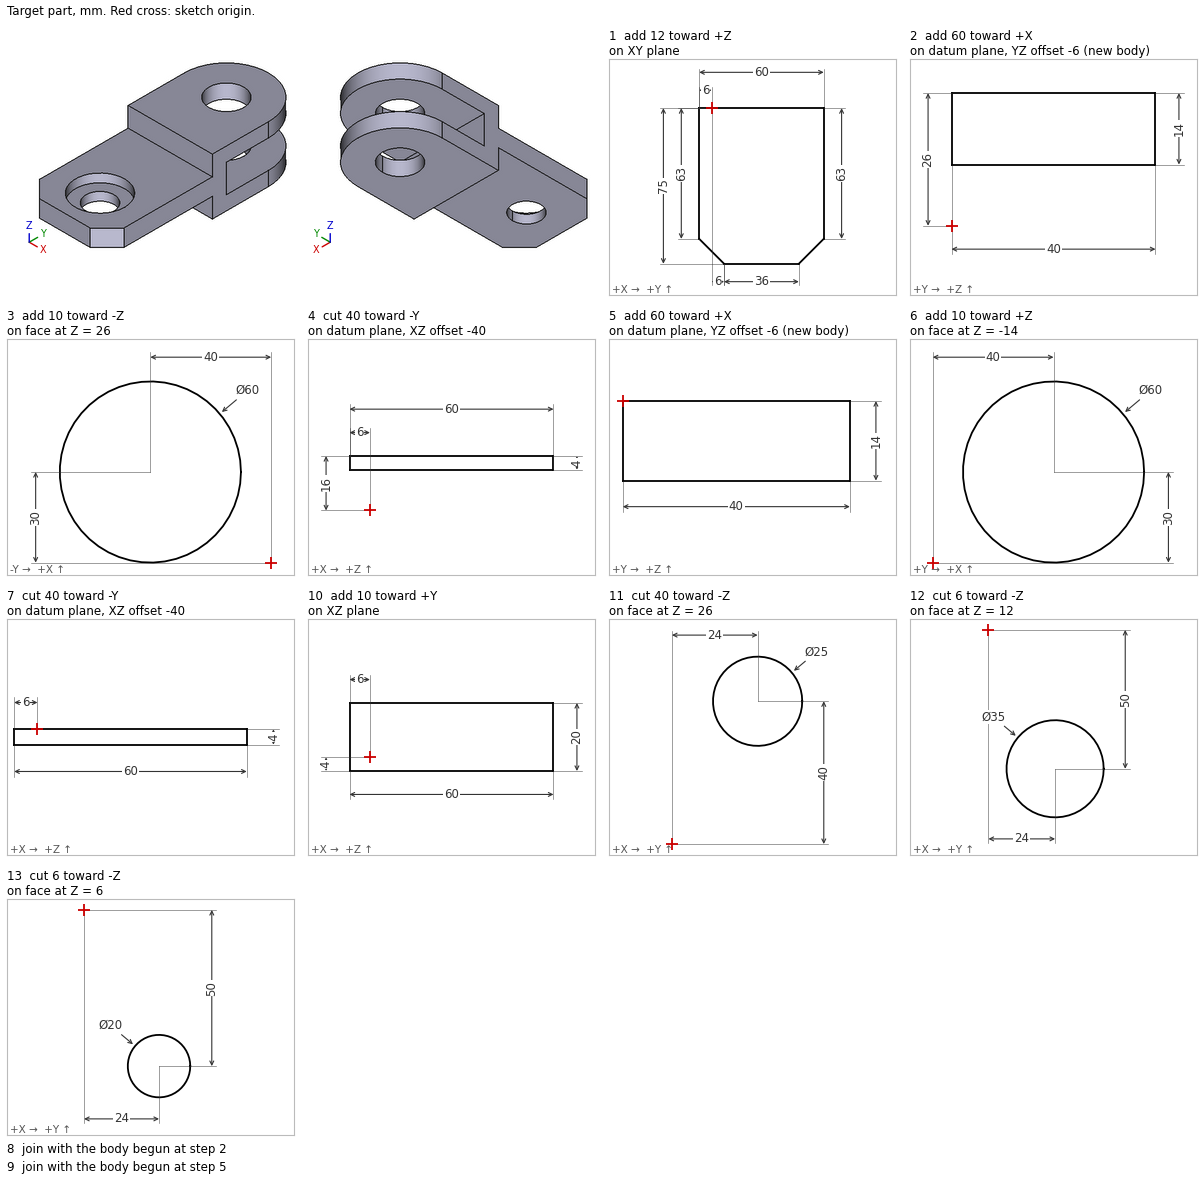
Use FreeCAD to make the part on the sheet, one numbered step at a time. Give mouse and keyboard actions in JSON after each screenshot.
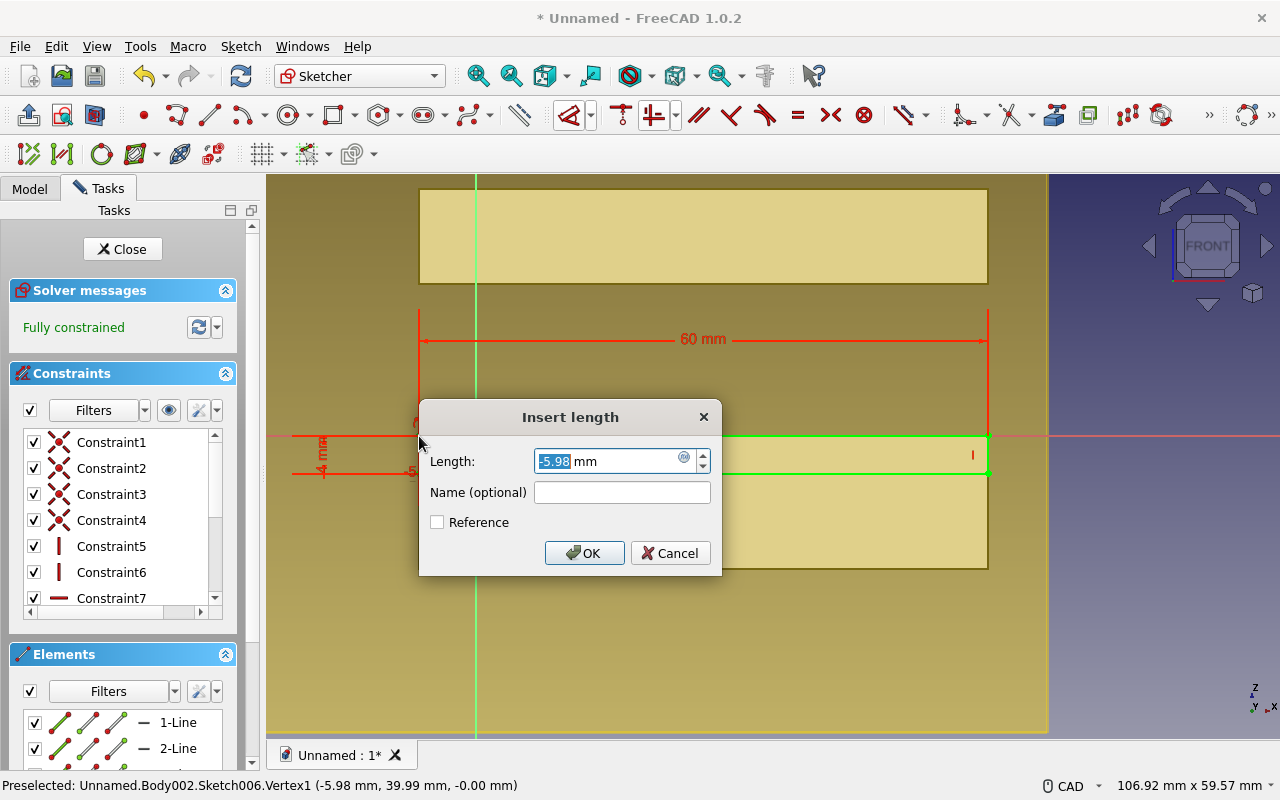
{"action": "type", "text": "-6"}
{"action": "key", "text": "Return"}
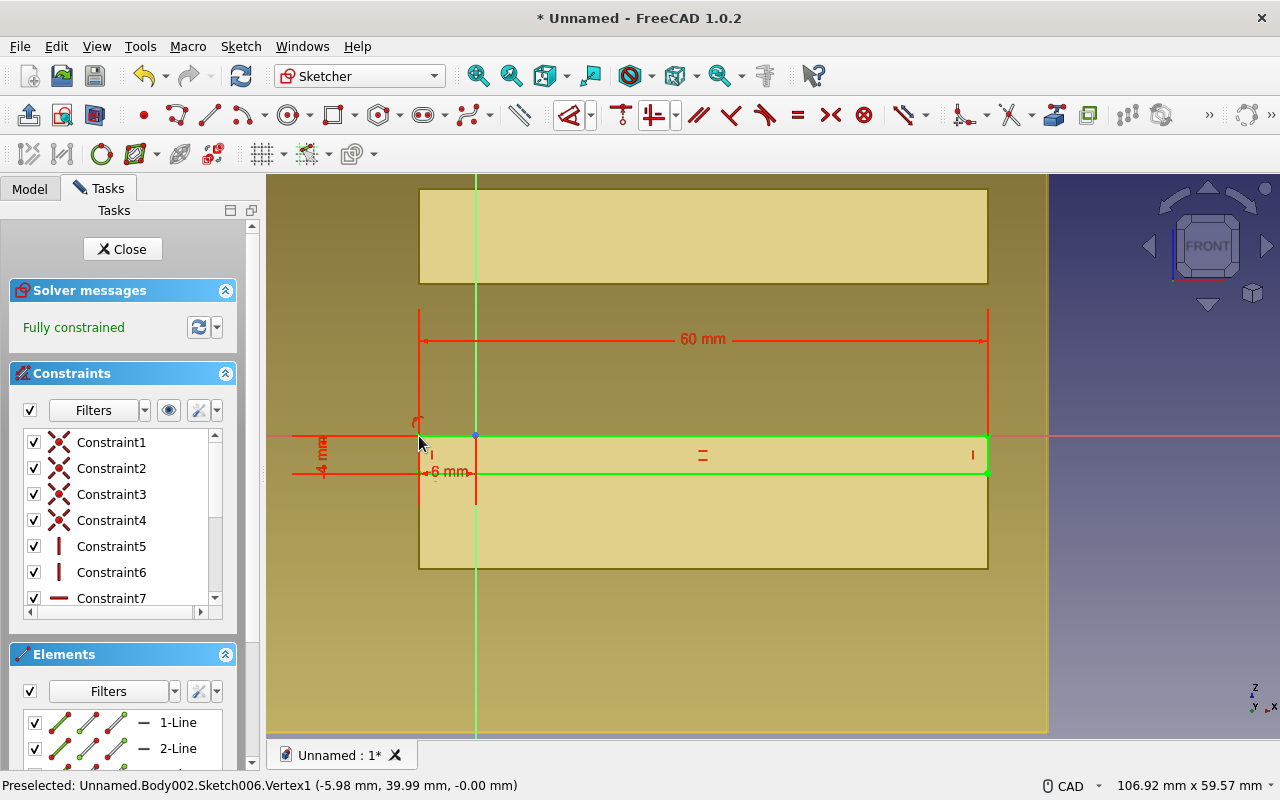
{"action": "left_click", "coordinate": [123, 249]}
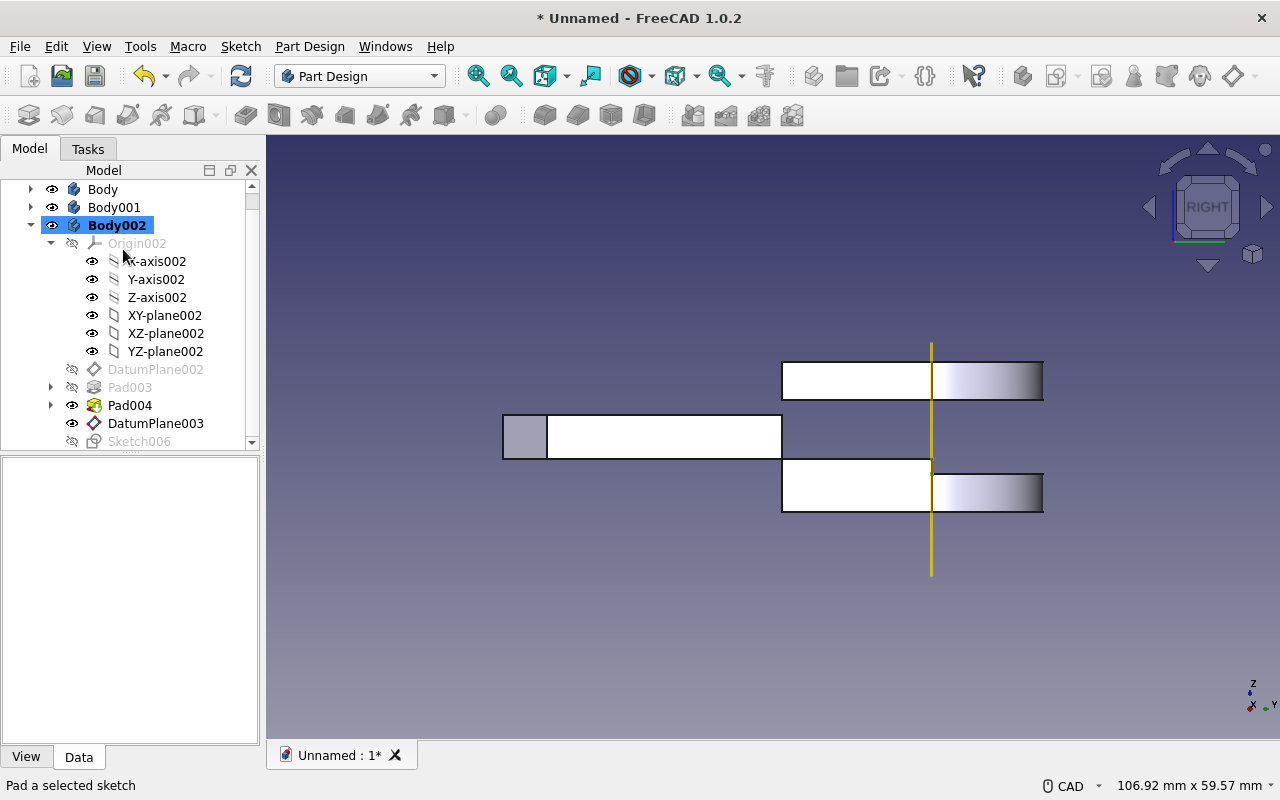
{"action": "left_click", "coordinate": [246, 116]}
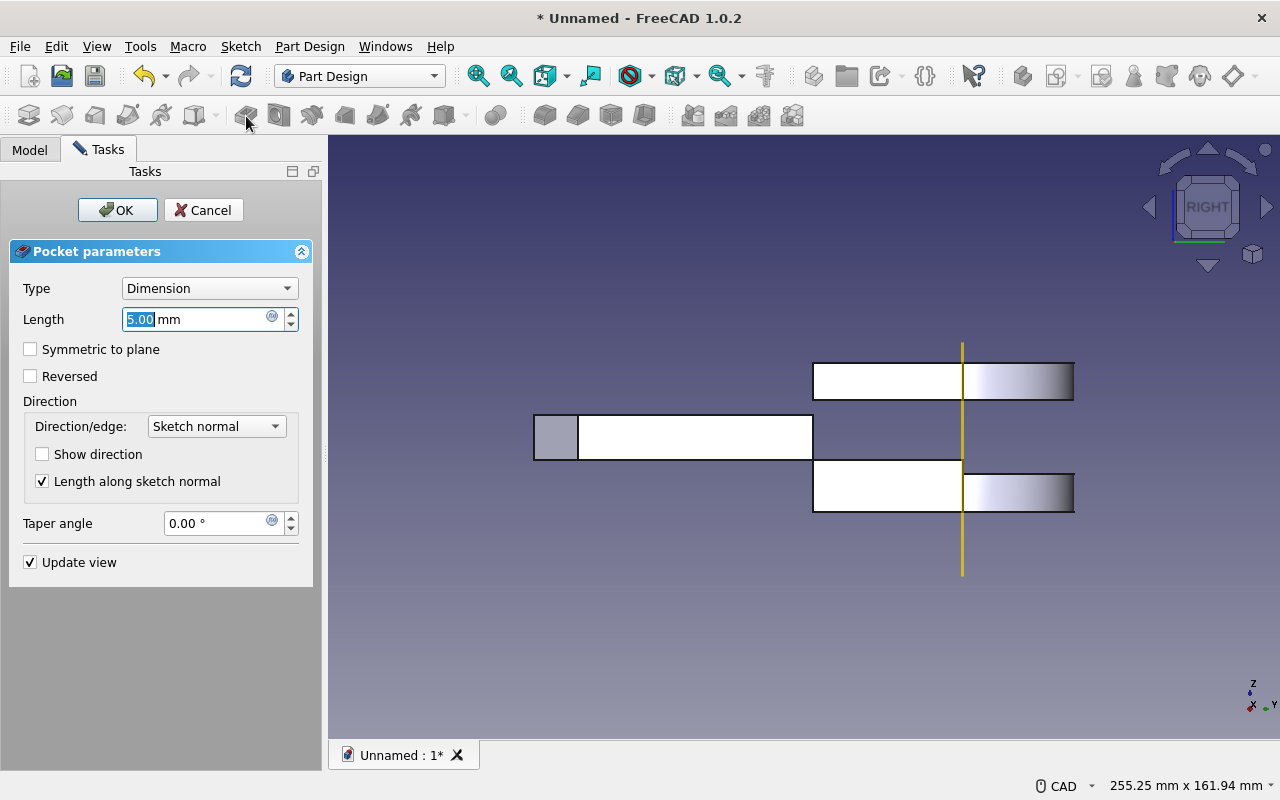
{"action": "type", "text": "40"}
{"action": "key", "text": "Tab"}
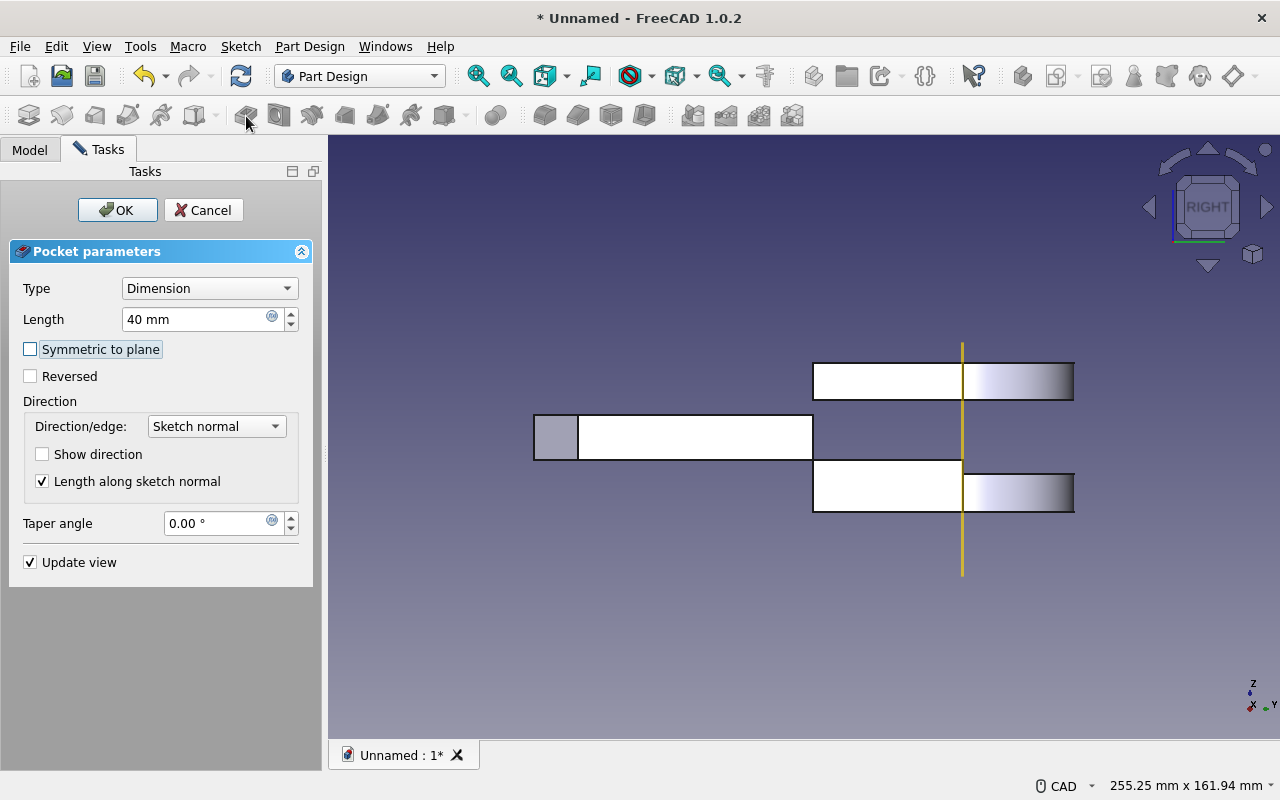
{"action": "left_click", "coordinate": [31, 376]}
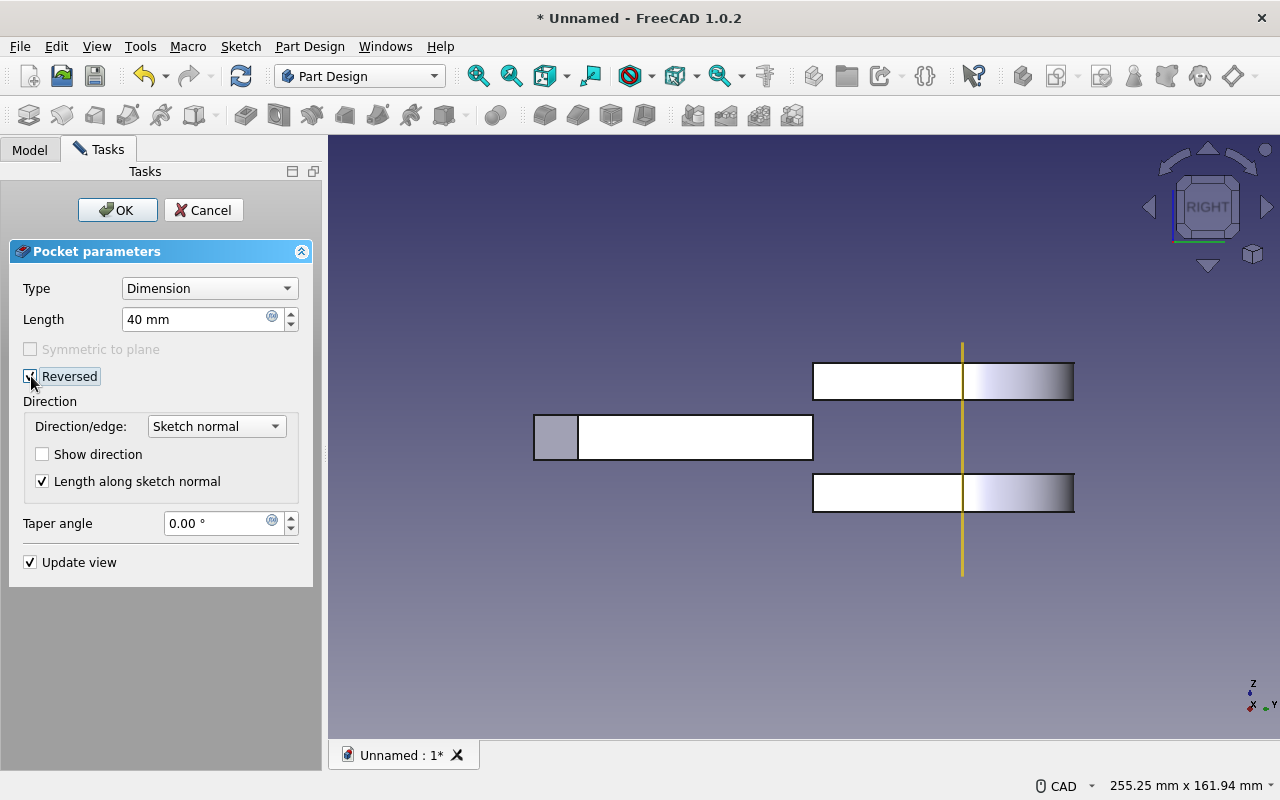
{"action": "left_click", "coordinate": [118, 210]}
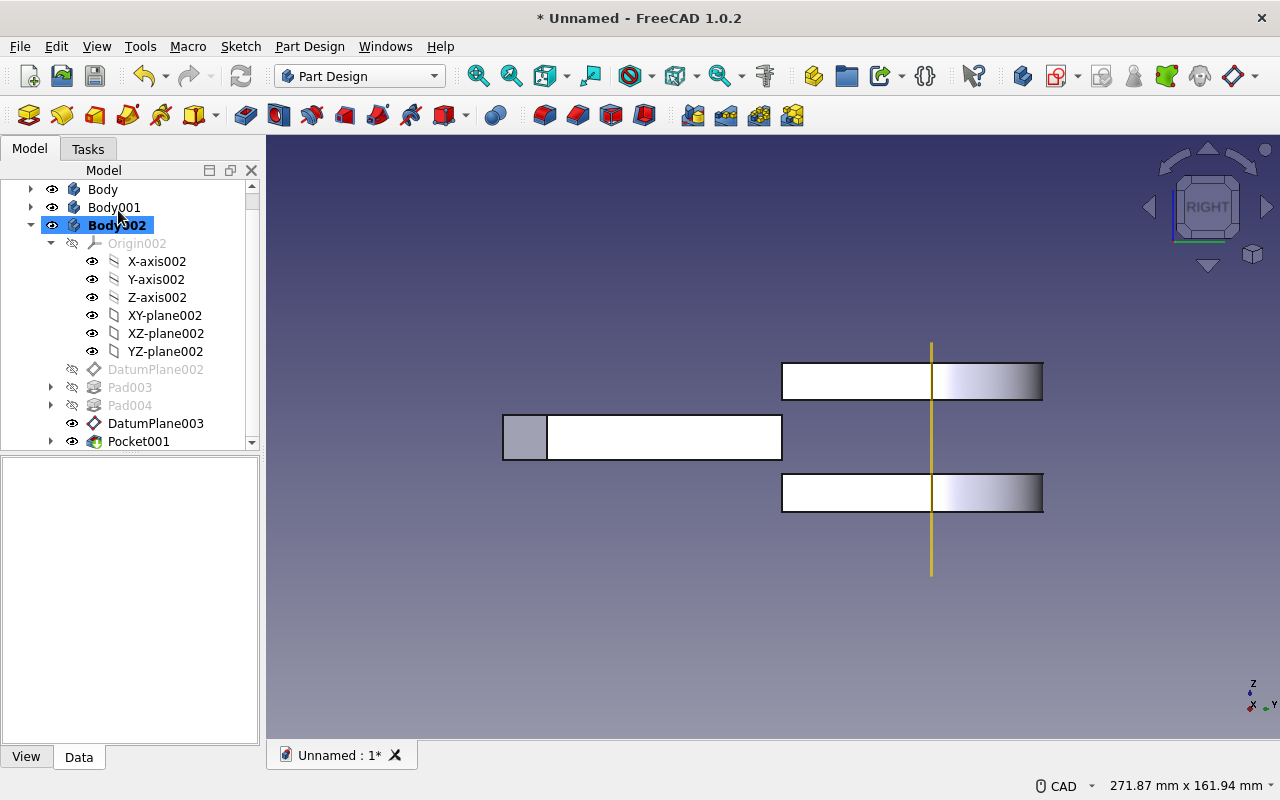
{"action": "left_click", "coordinate": [117, 423]}
{"action": "key", "text": "space"}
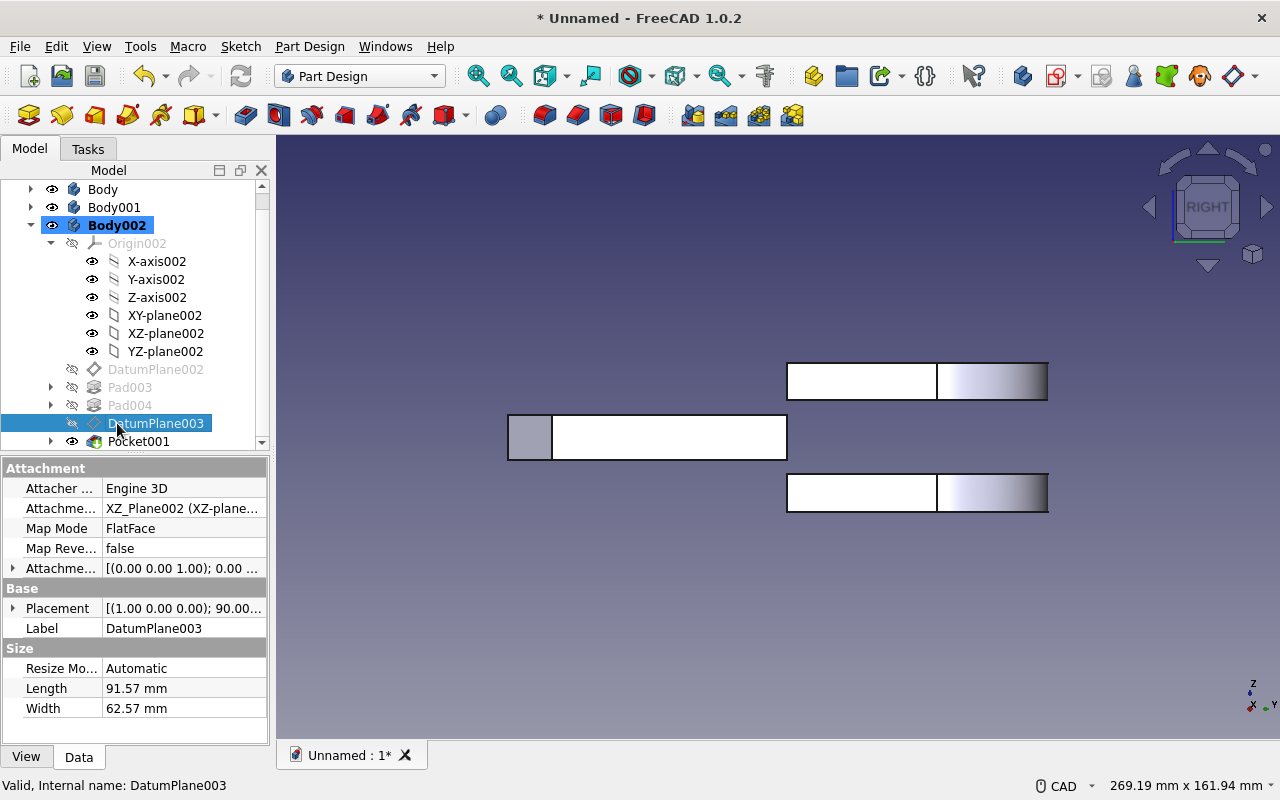
{"action": "left_click", "coordinate": [479, 76]}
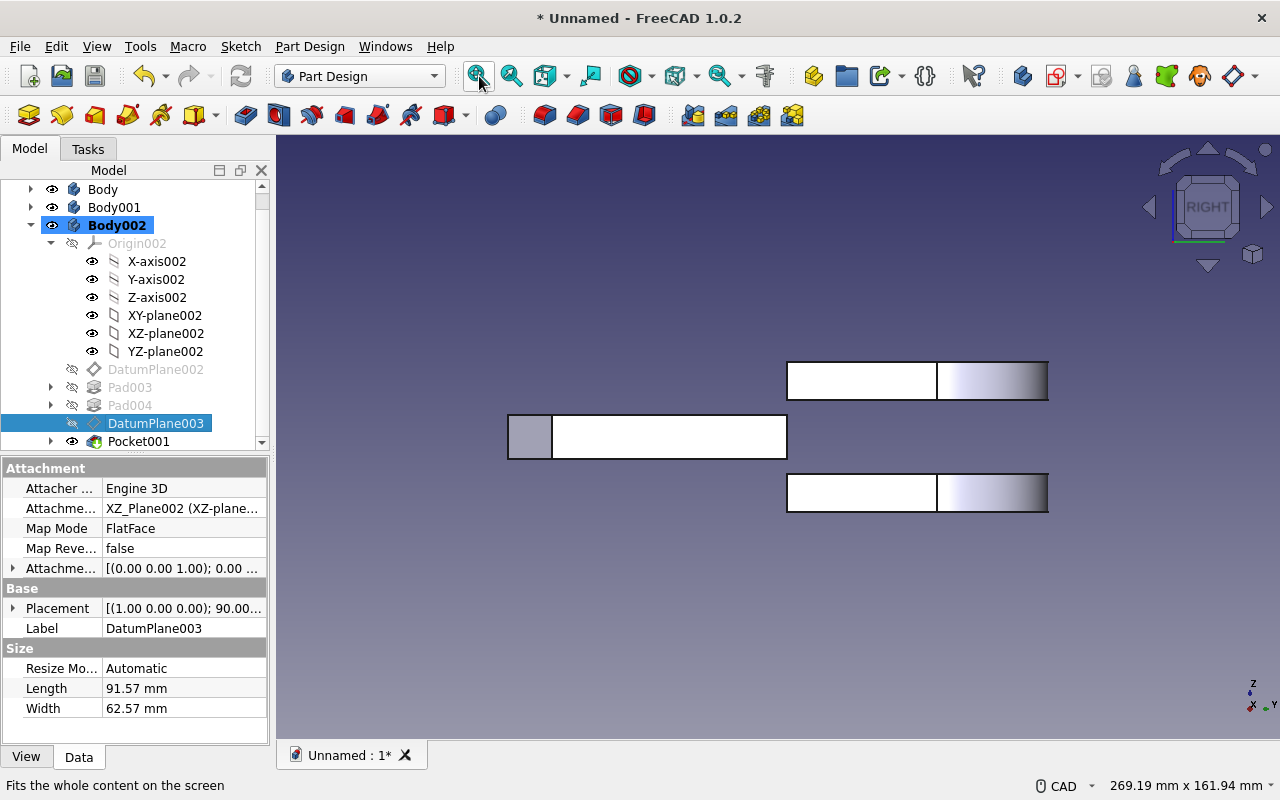
{"action": "double_click", "coordinate": [97, 189]}